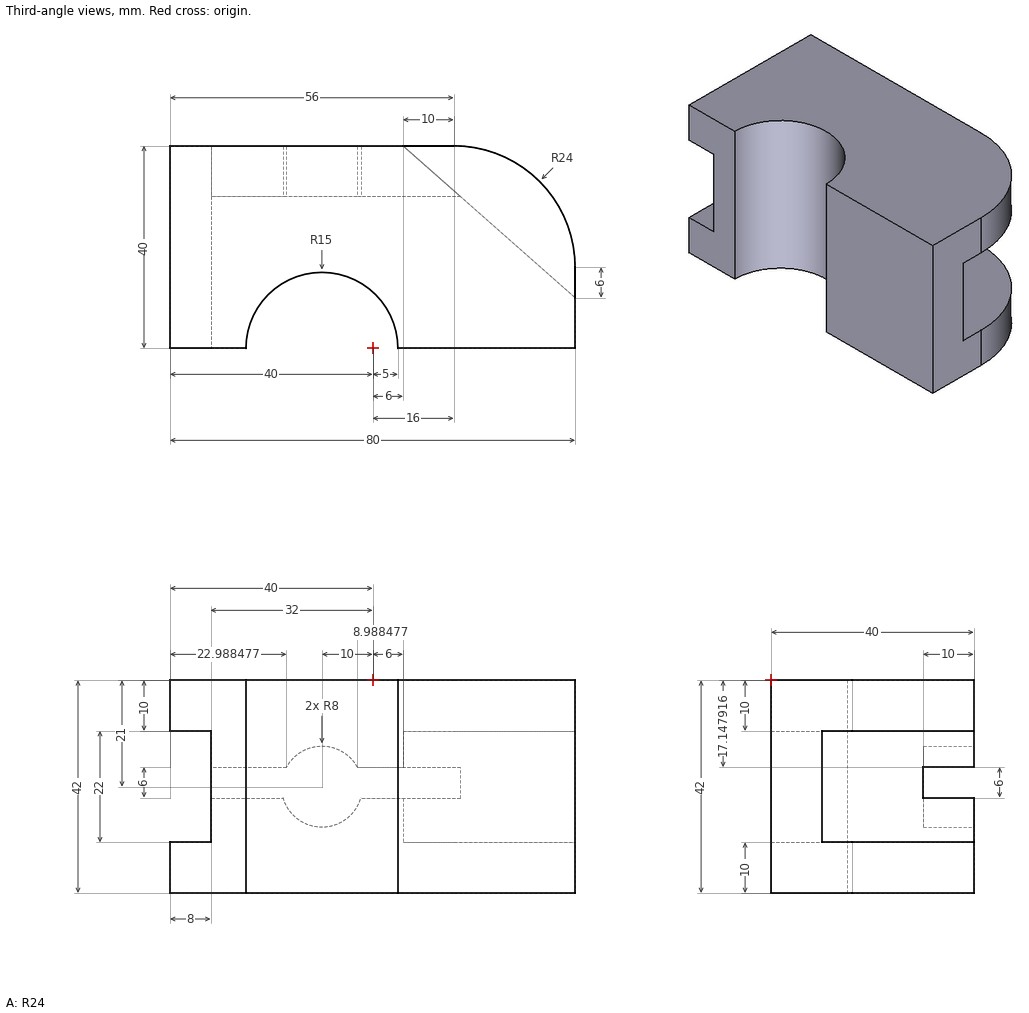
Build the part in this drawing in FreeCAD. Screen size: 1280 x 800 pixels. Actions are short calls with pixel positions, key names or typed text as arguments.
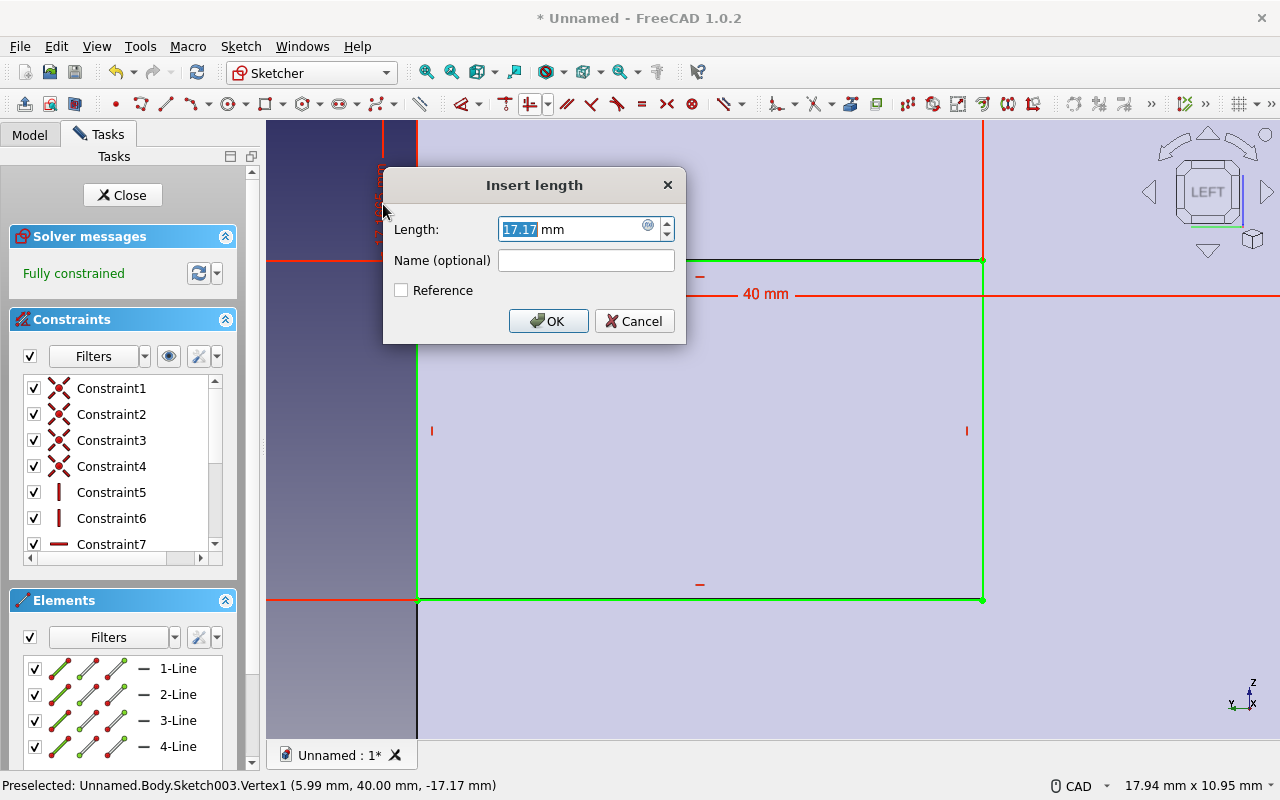
text(17.147916)
key(Return)
key(Escape)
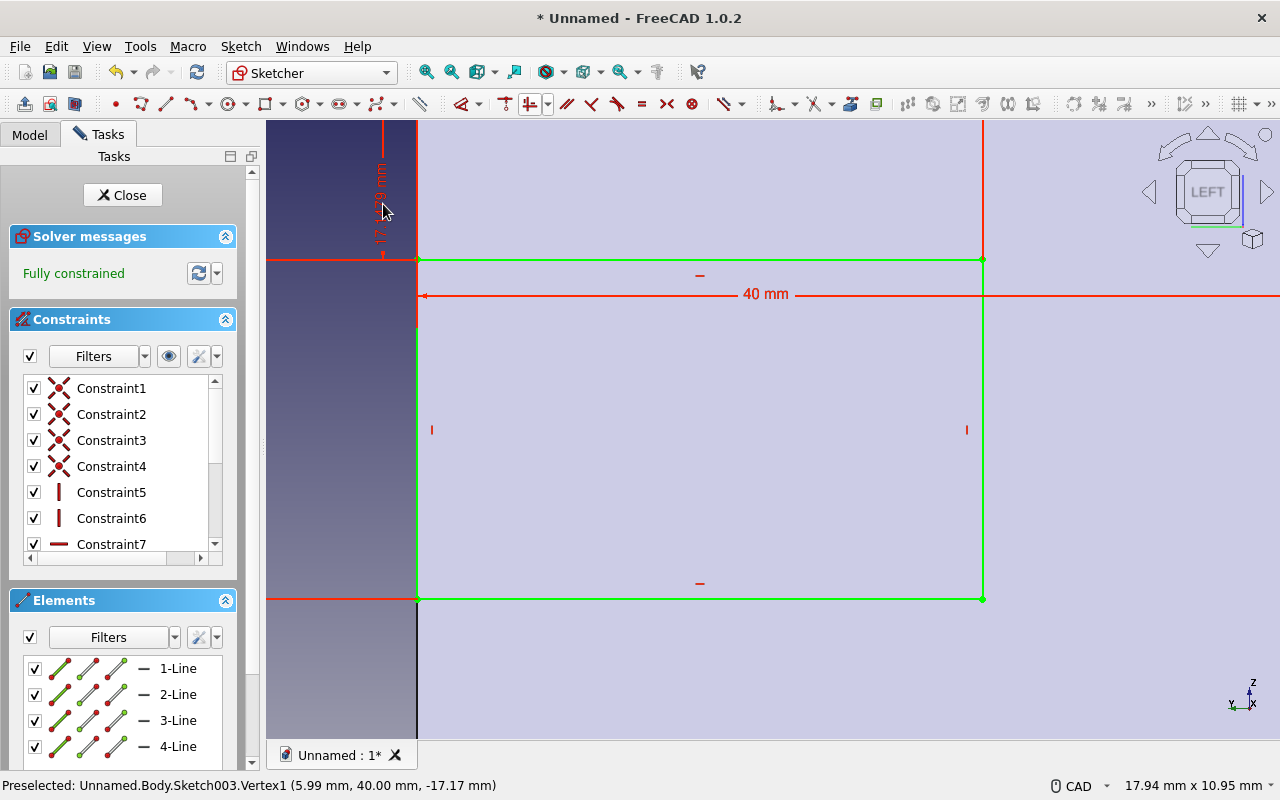
click(123, 195)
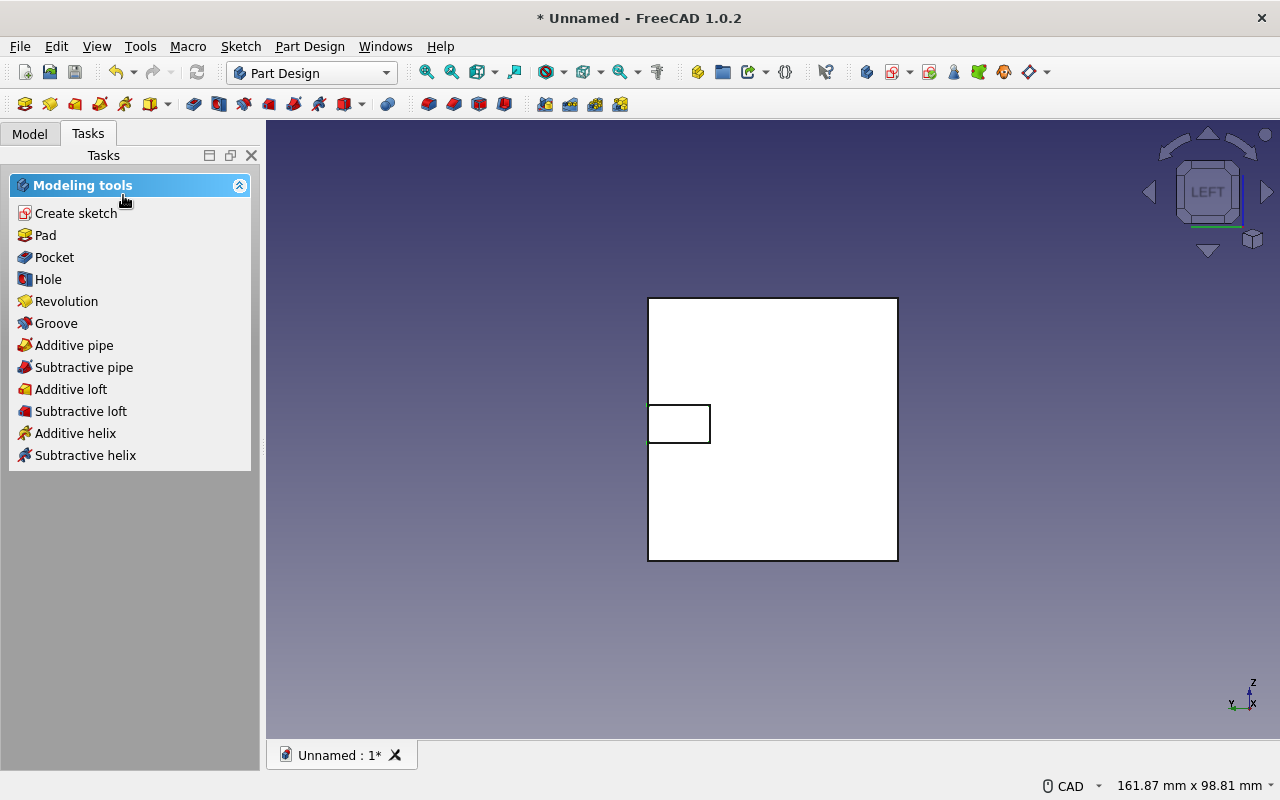
click(194, 104)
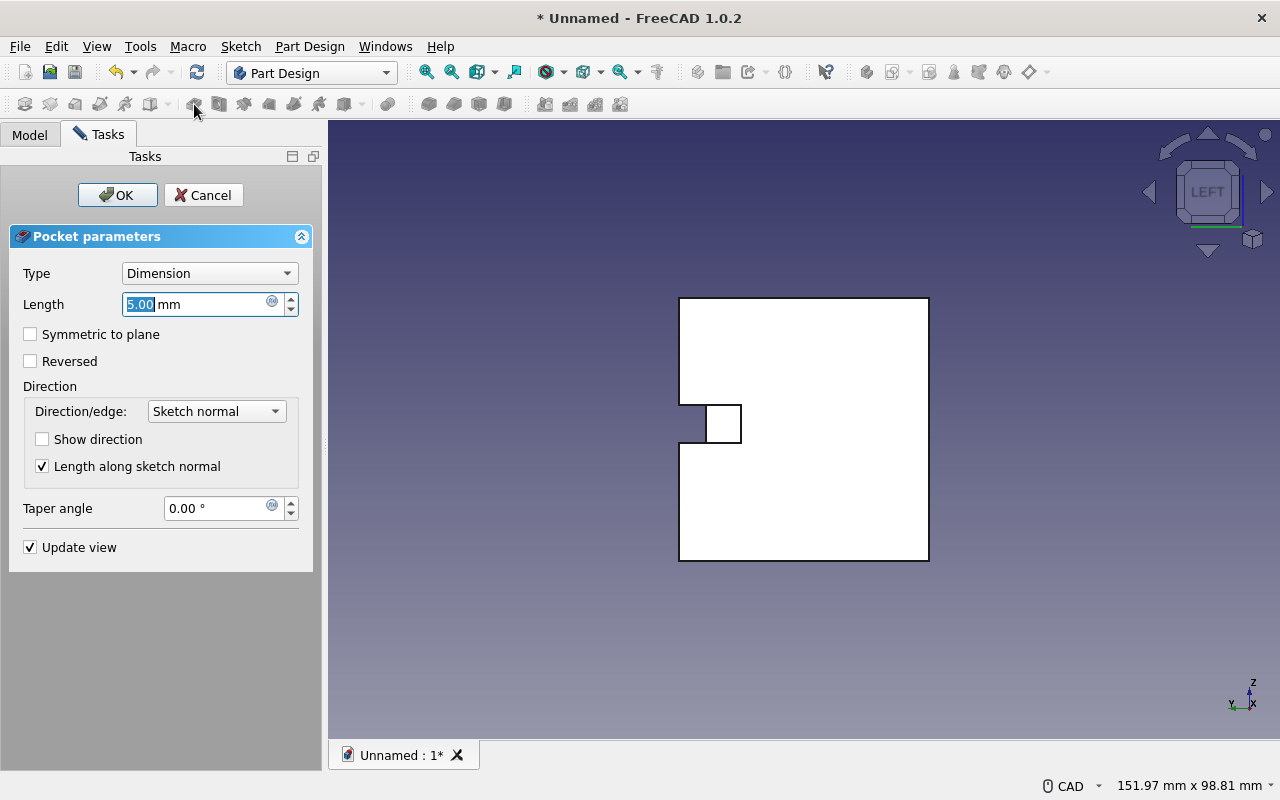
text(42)
key(Tab)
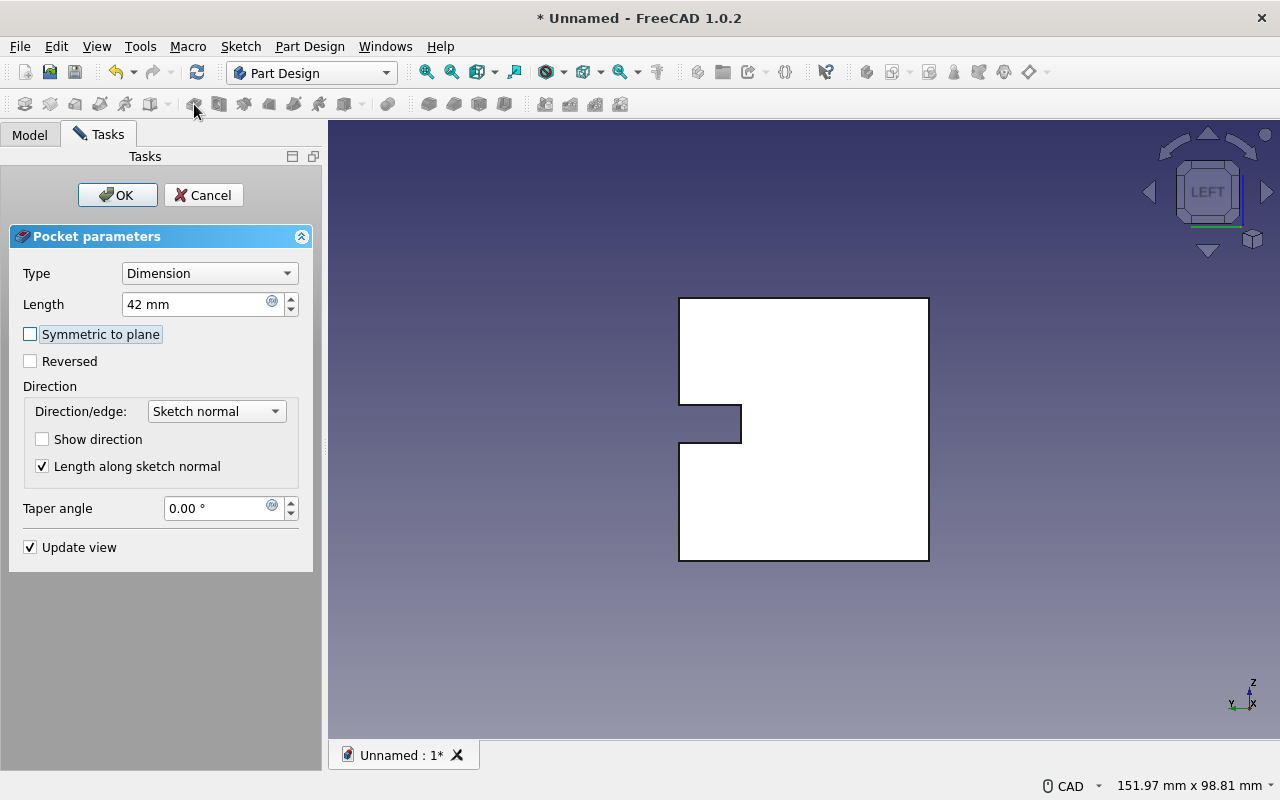
click(118, 195)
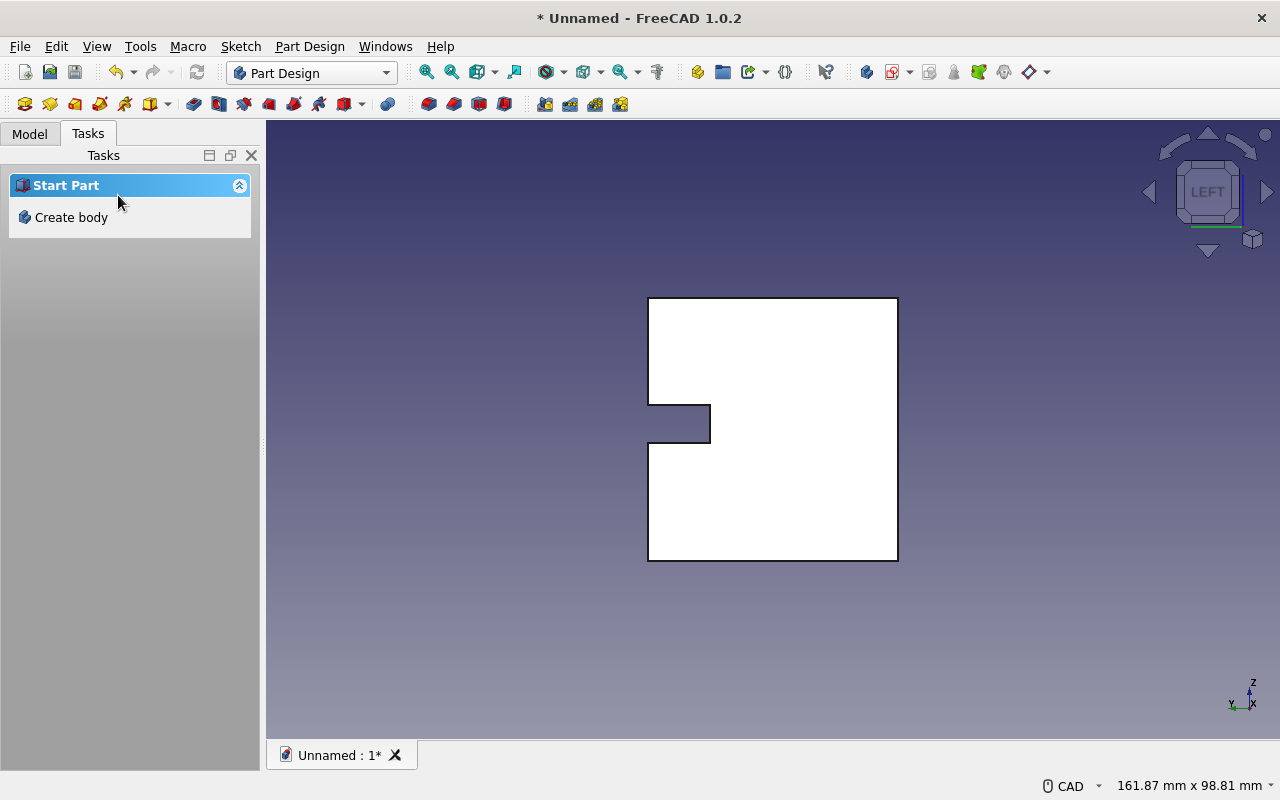
key(v)
key(f)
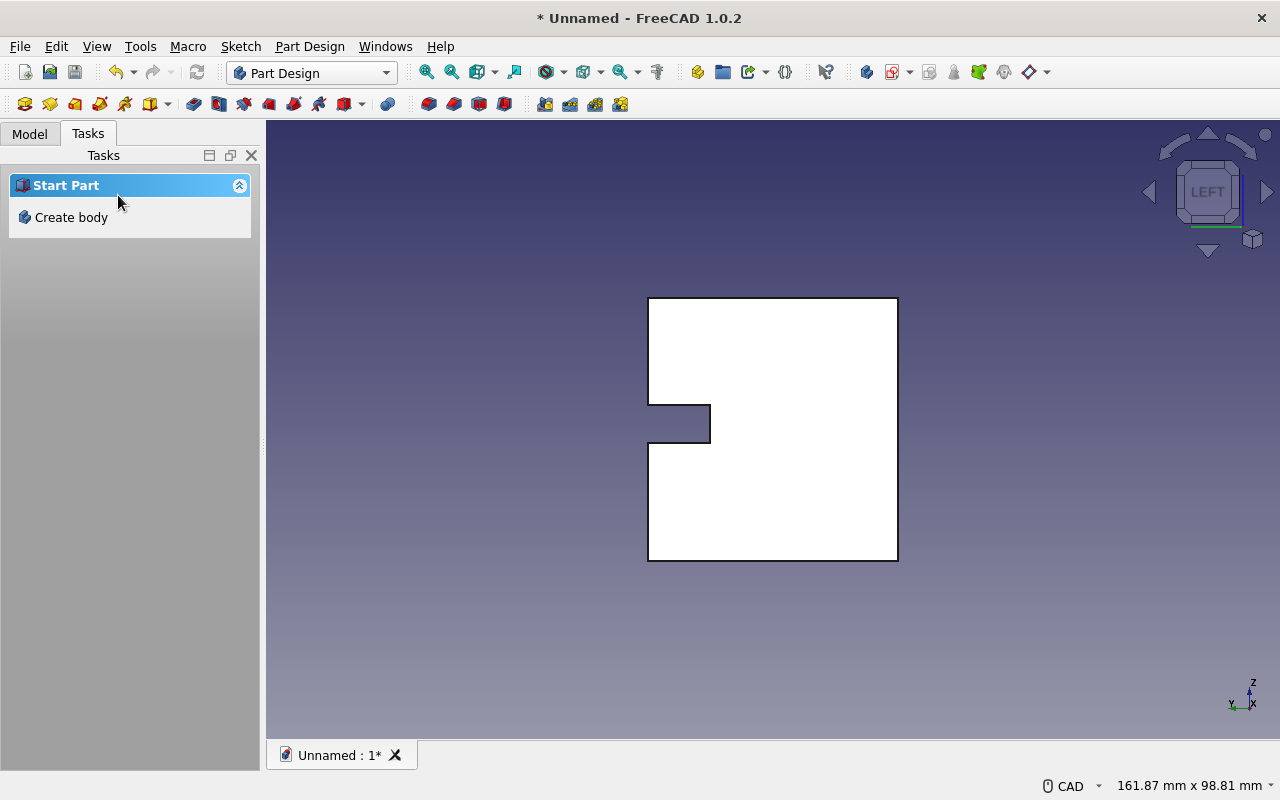
key(0)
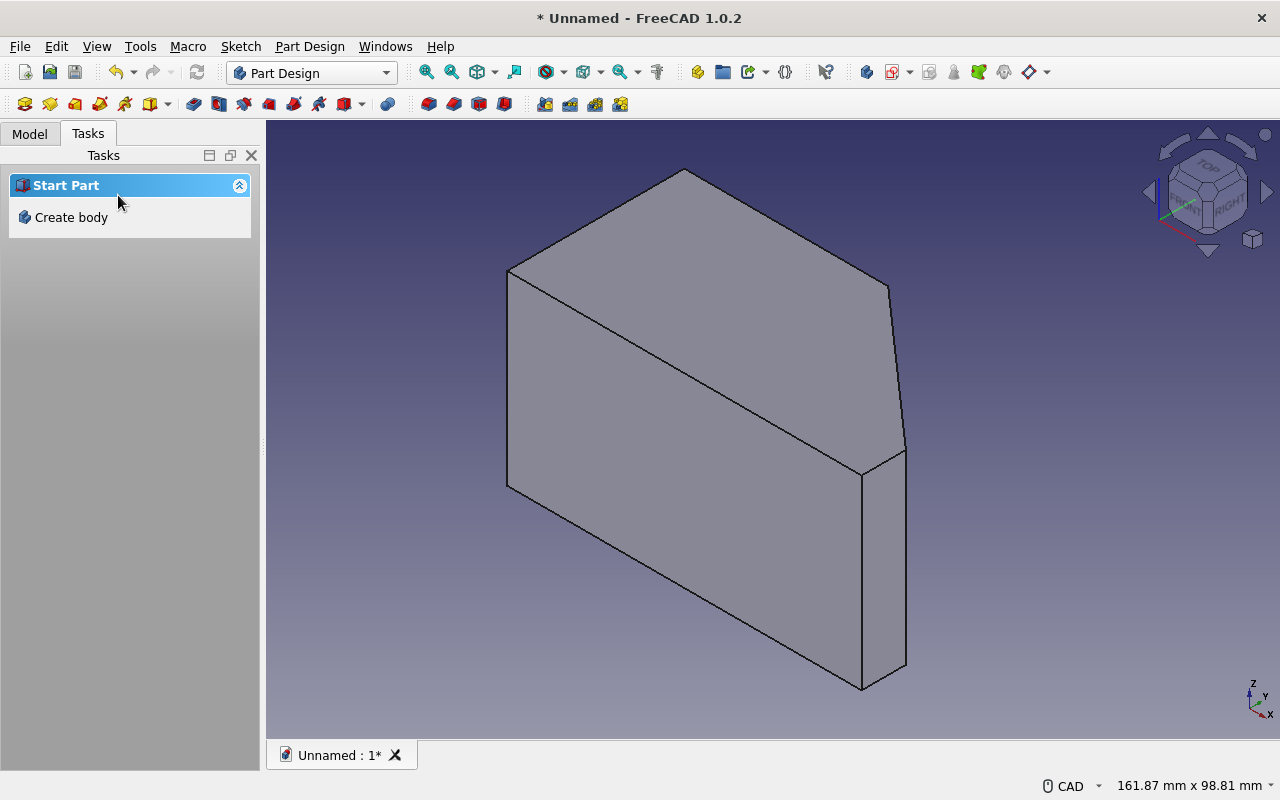
click(722, 292)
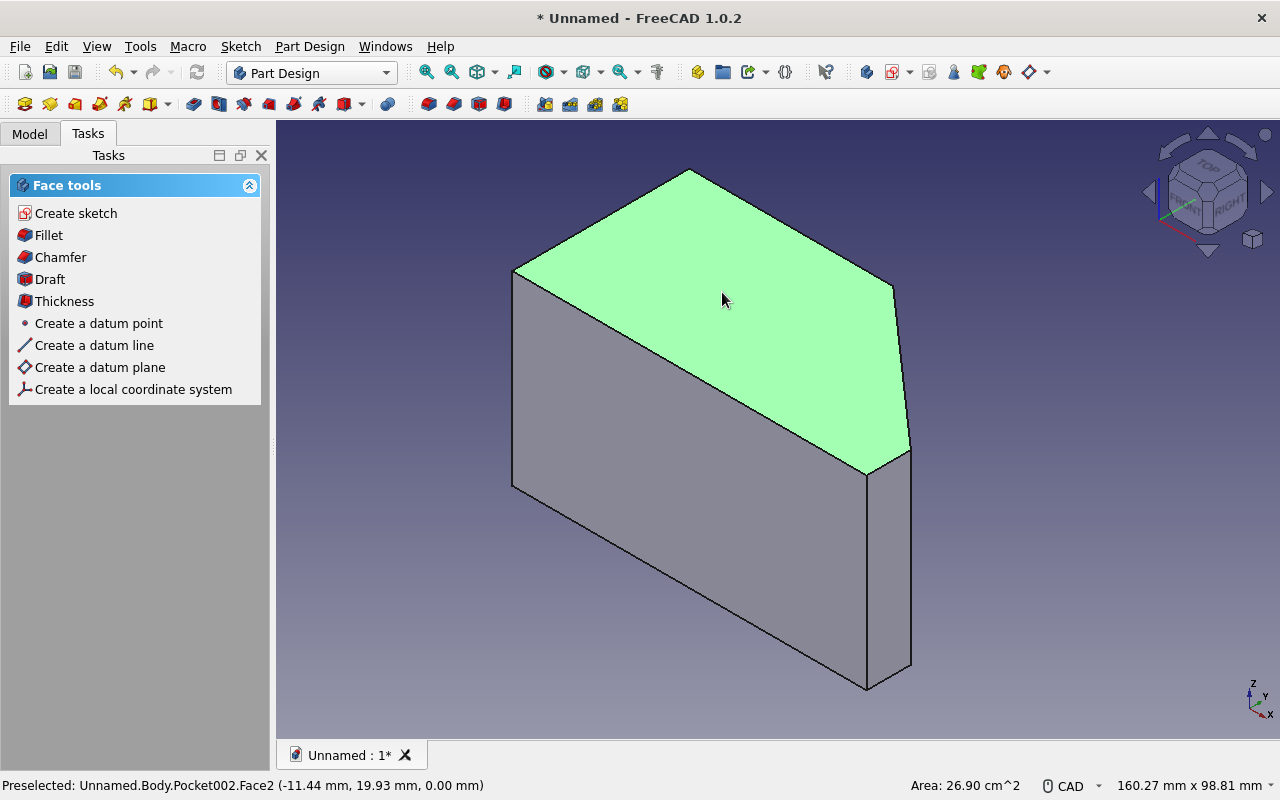
click(892, 72)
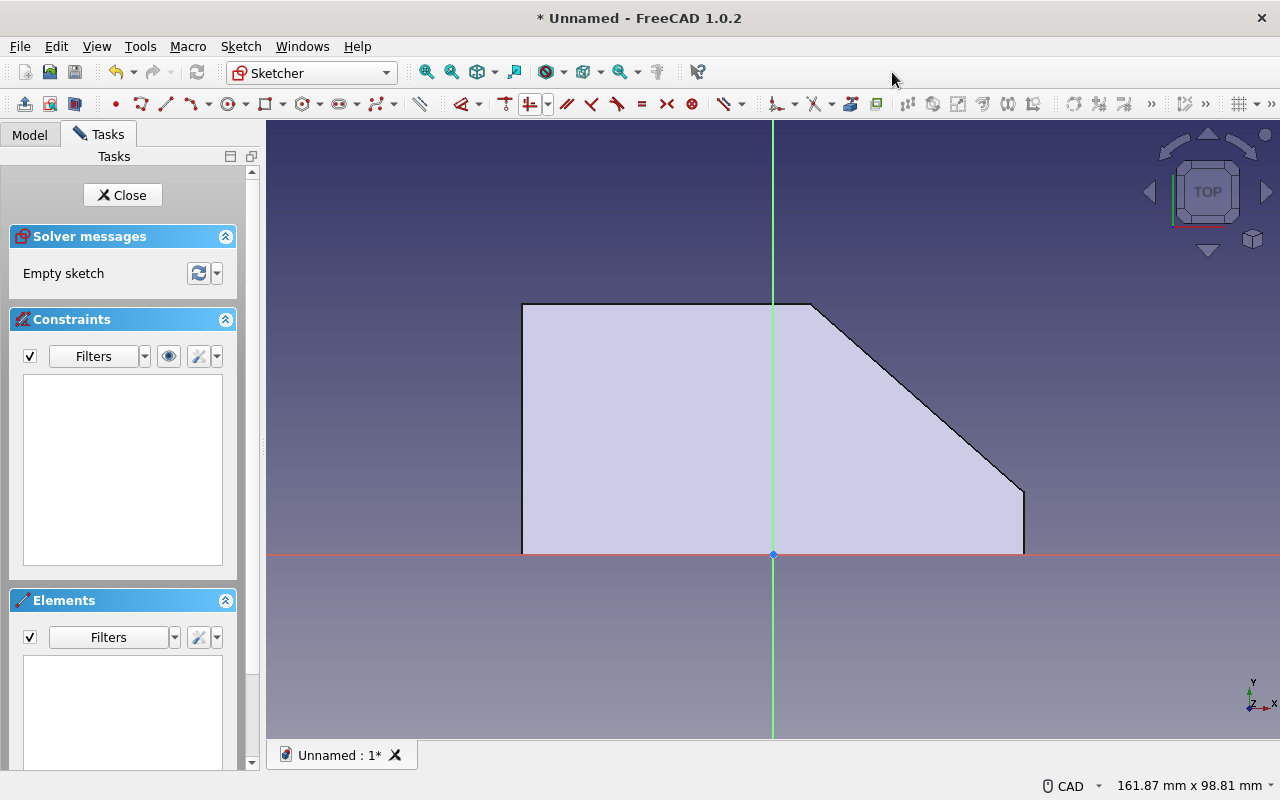
key(g)
key(r)